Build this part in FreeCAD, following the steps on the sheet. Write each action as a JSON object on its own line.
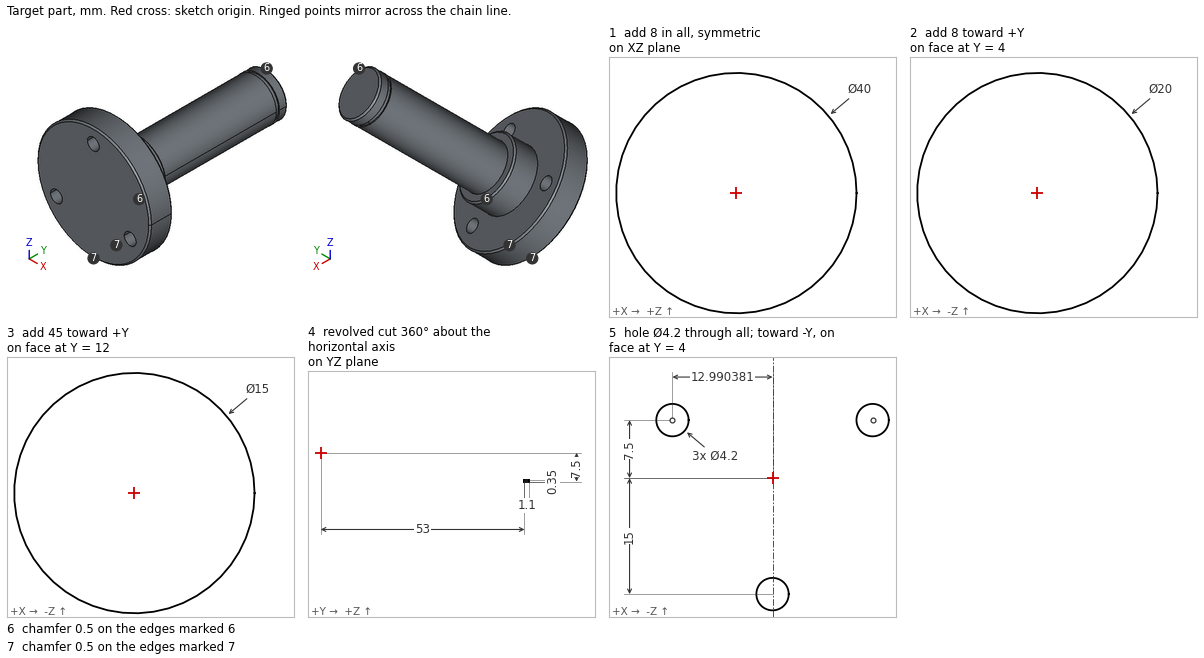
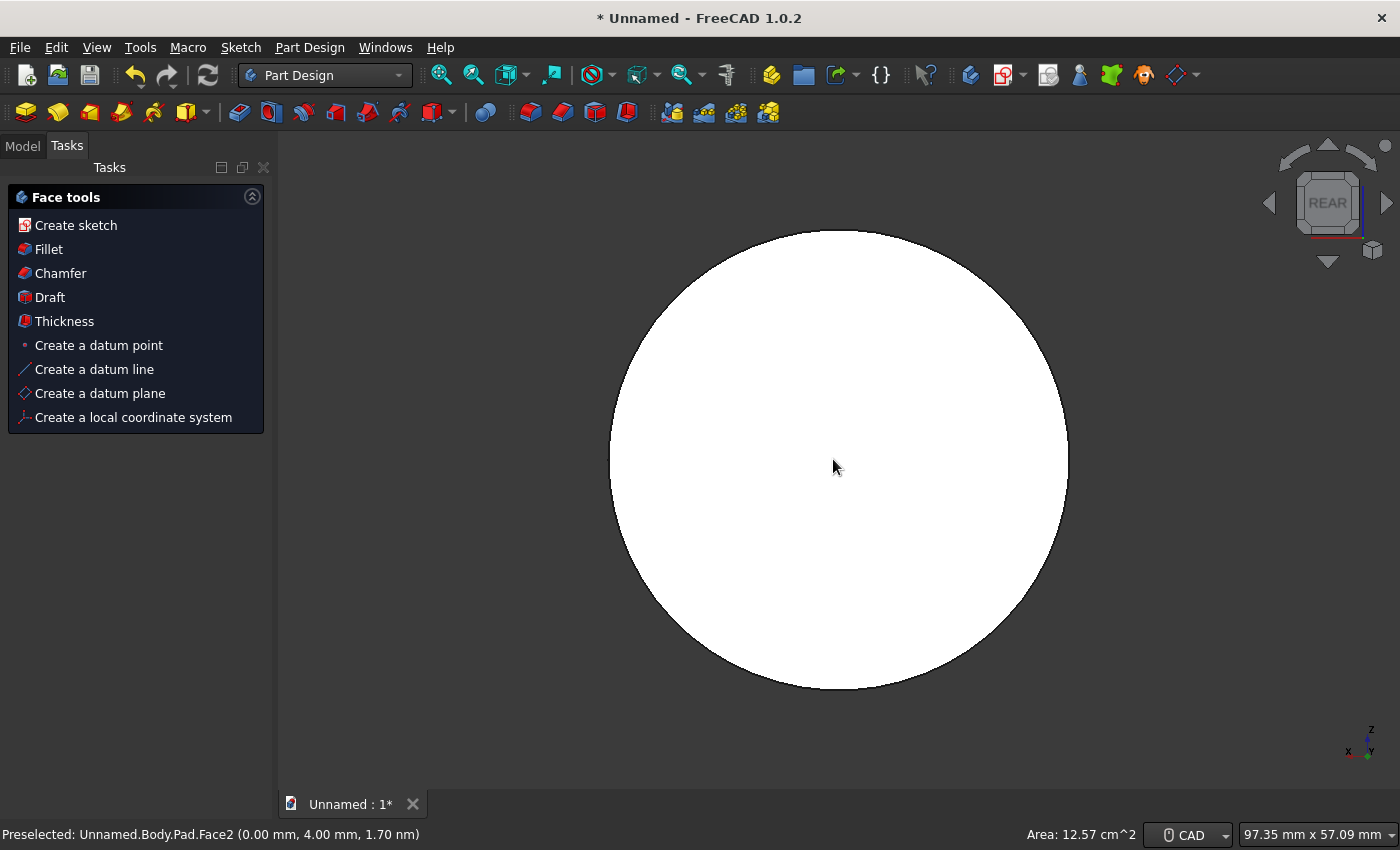
{"action": "left_click", "coordinate": [1004, 76]}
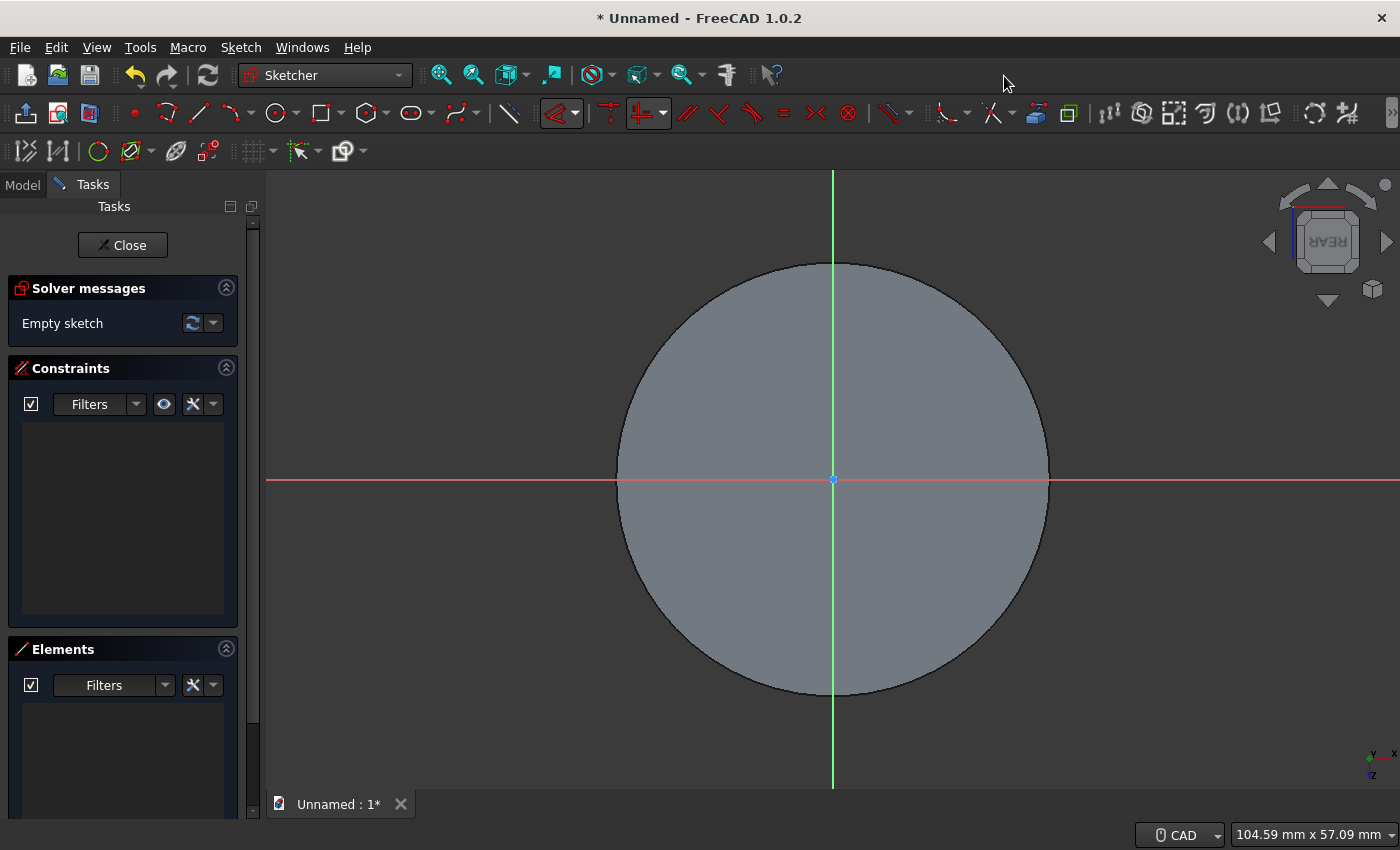
{"action": "scroll", "coordinate": [916, 479], "scroll_direction": "up", "scroll_amount": 3}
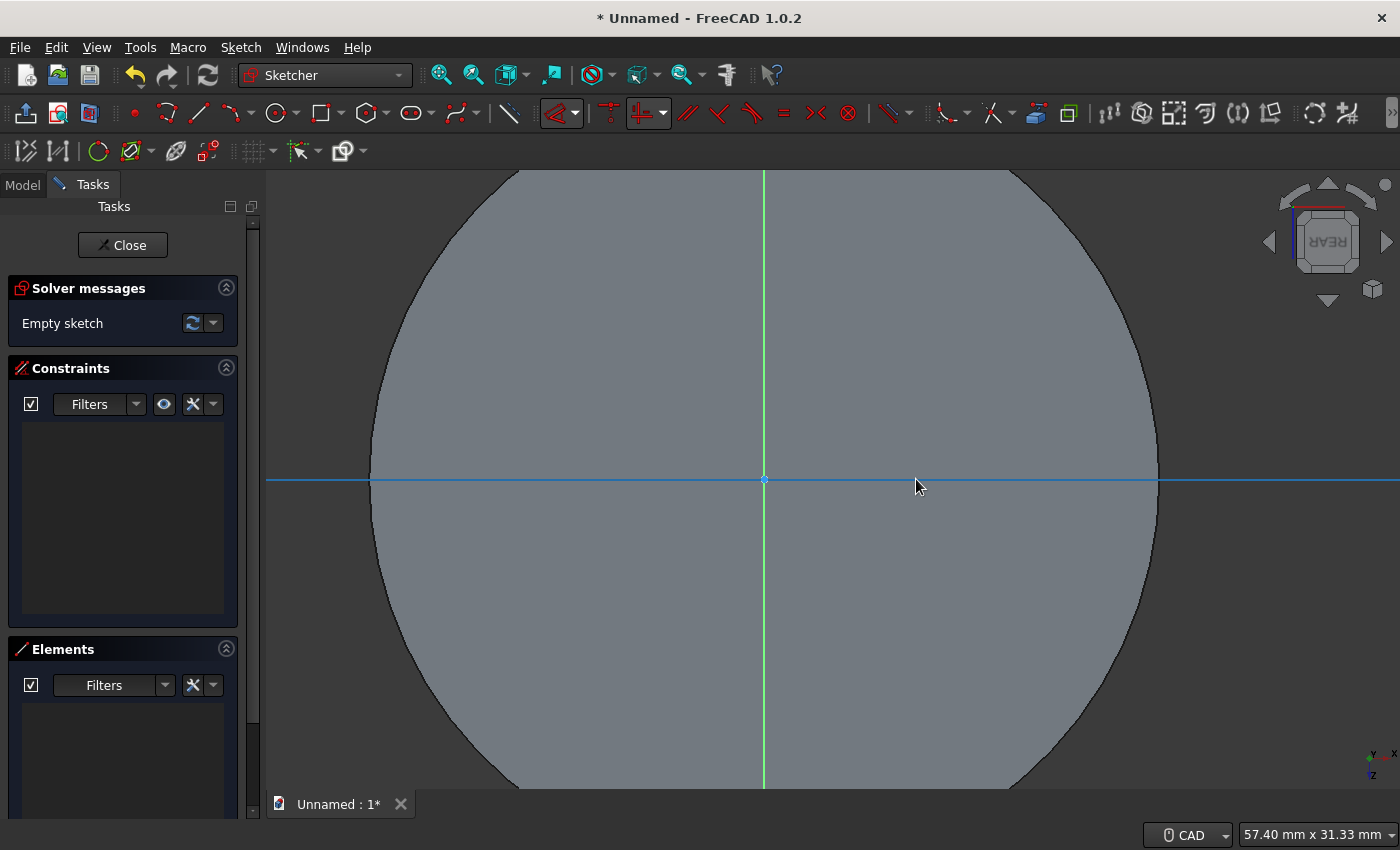
{"action": "left_click", "coordinate": [276, 114]}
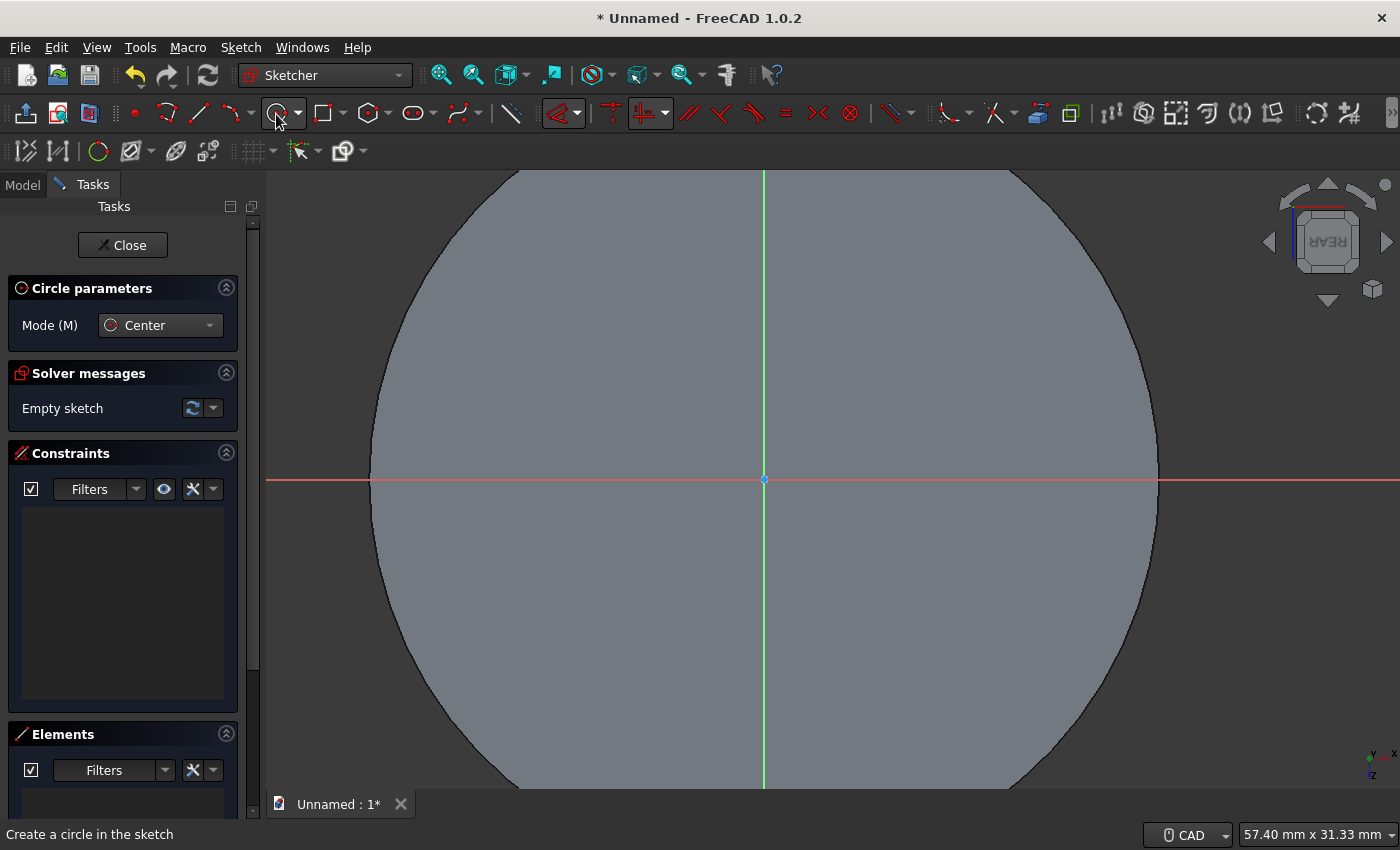
{"action": "left_click", "coordinate": [764, 479]}
{"action": "mouse_move", "coordinate": [904, 340]}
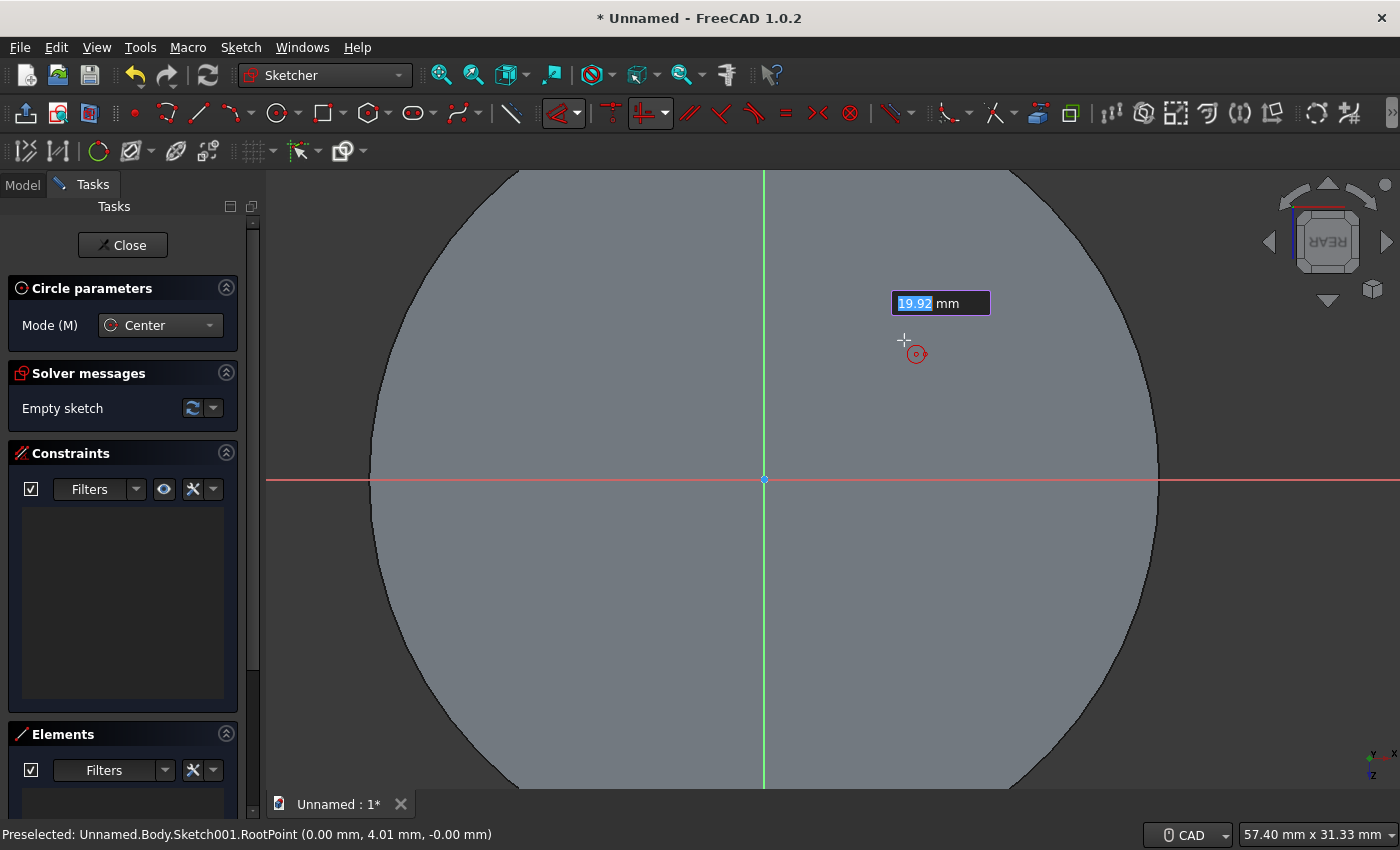
{"action": "type", "text": "20"}
{"action": "key", "text": "Return"}
{"action": "key", "text": "Escape"}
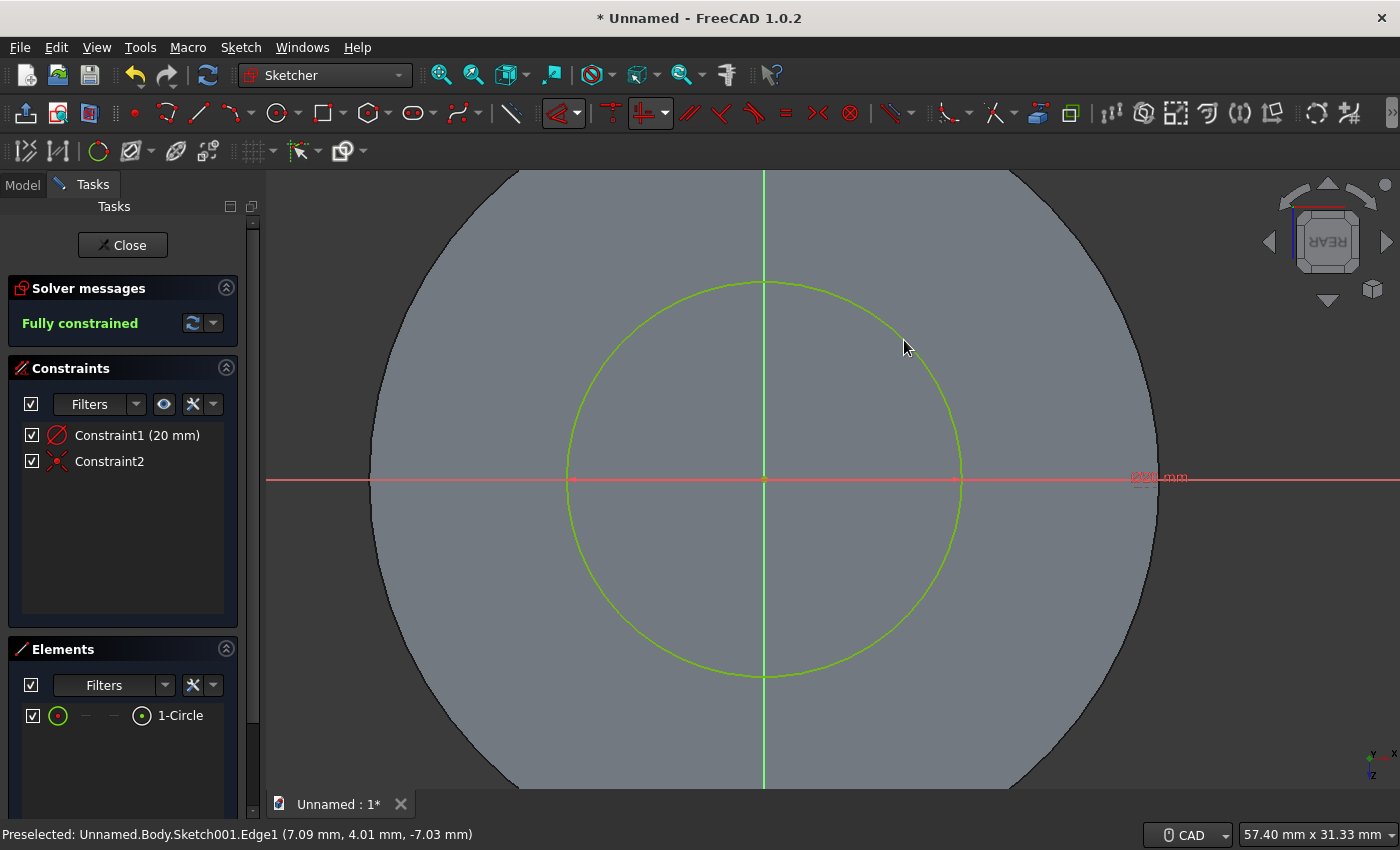
{"action": "left_click", "coordinate": [123, 245]}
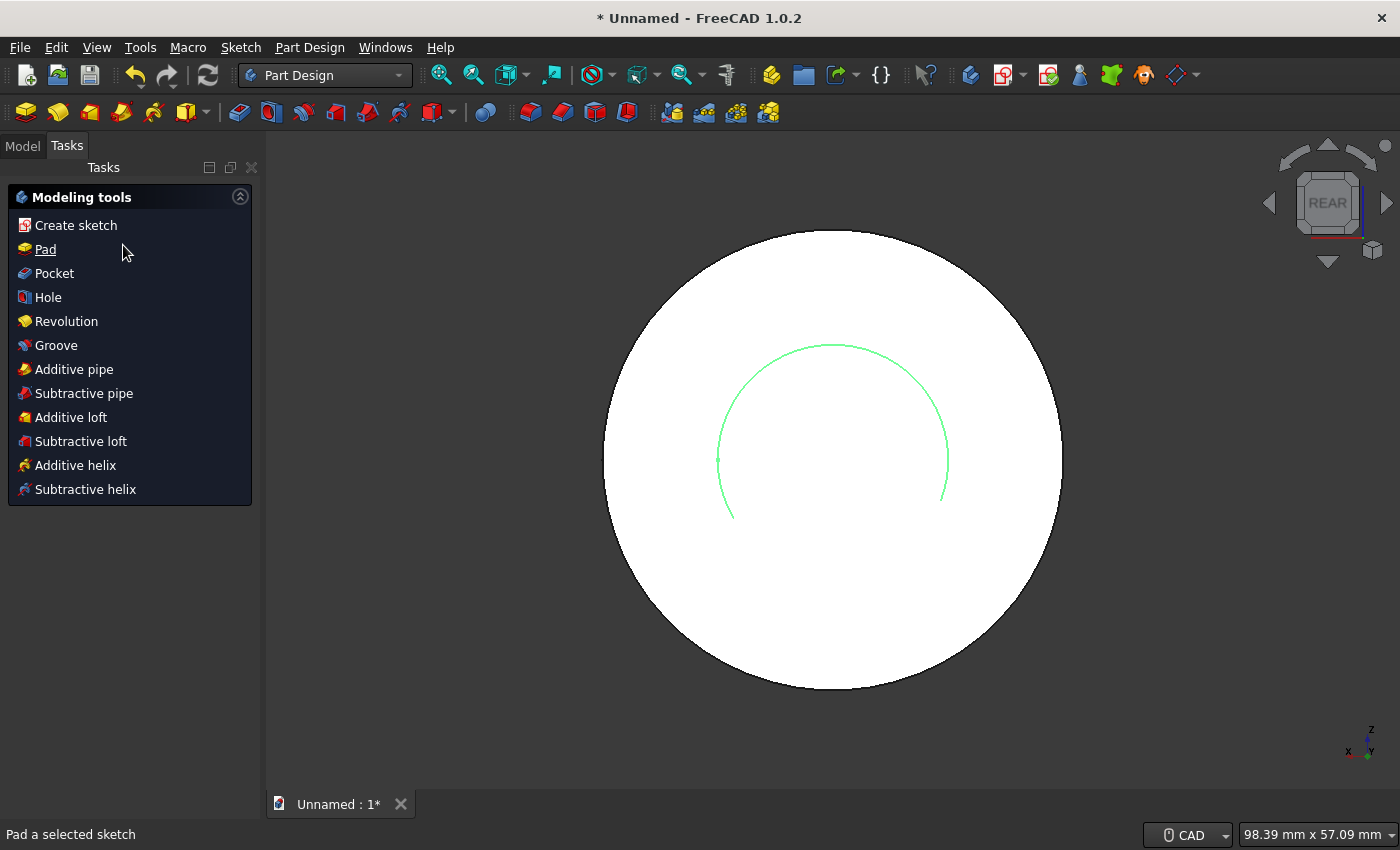
{"action": "left_click", "coordinate": [26, 112]}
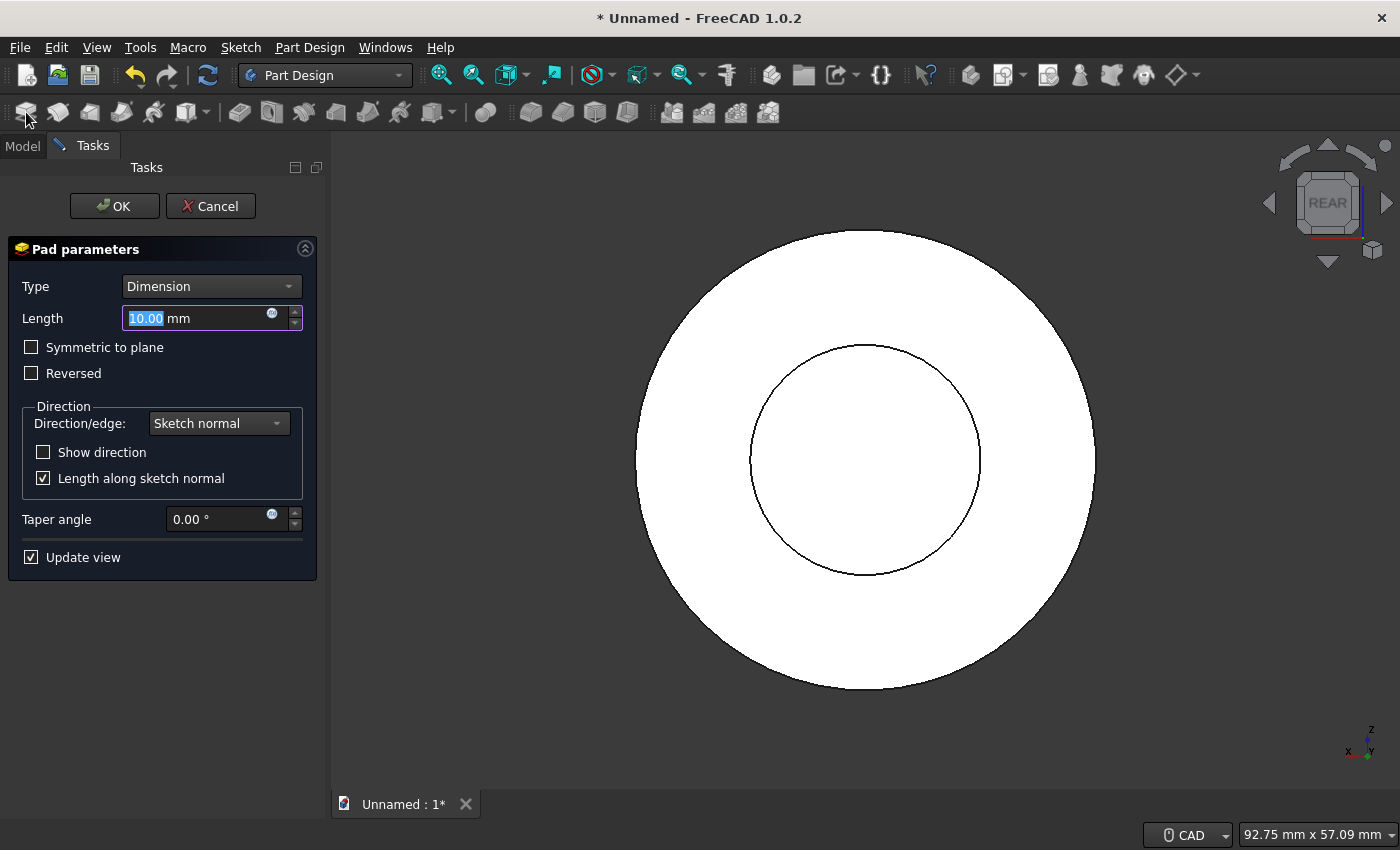
{"action": "type", "text": "8"}
{"action": "key", "text": "Tab"}